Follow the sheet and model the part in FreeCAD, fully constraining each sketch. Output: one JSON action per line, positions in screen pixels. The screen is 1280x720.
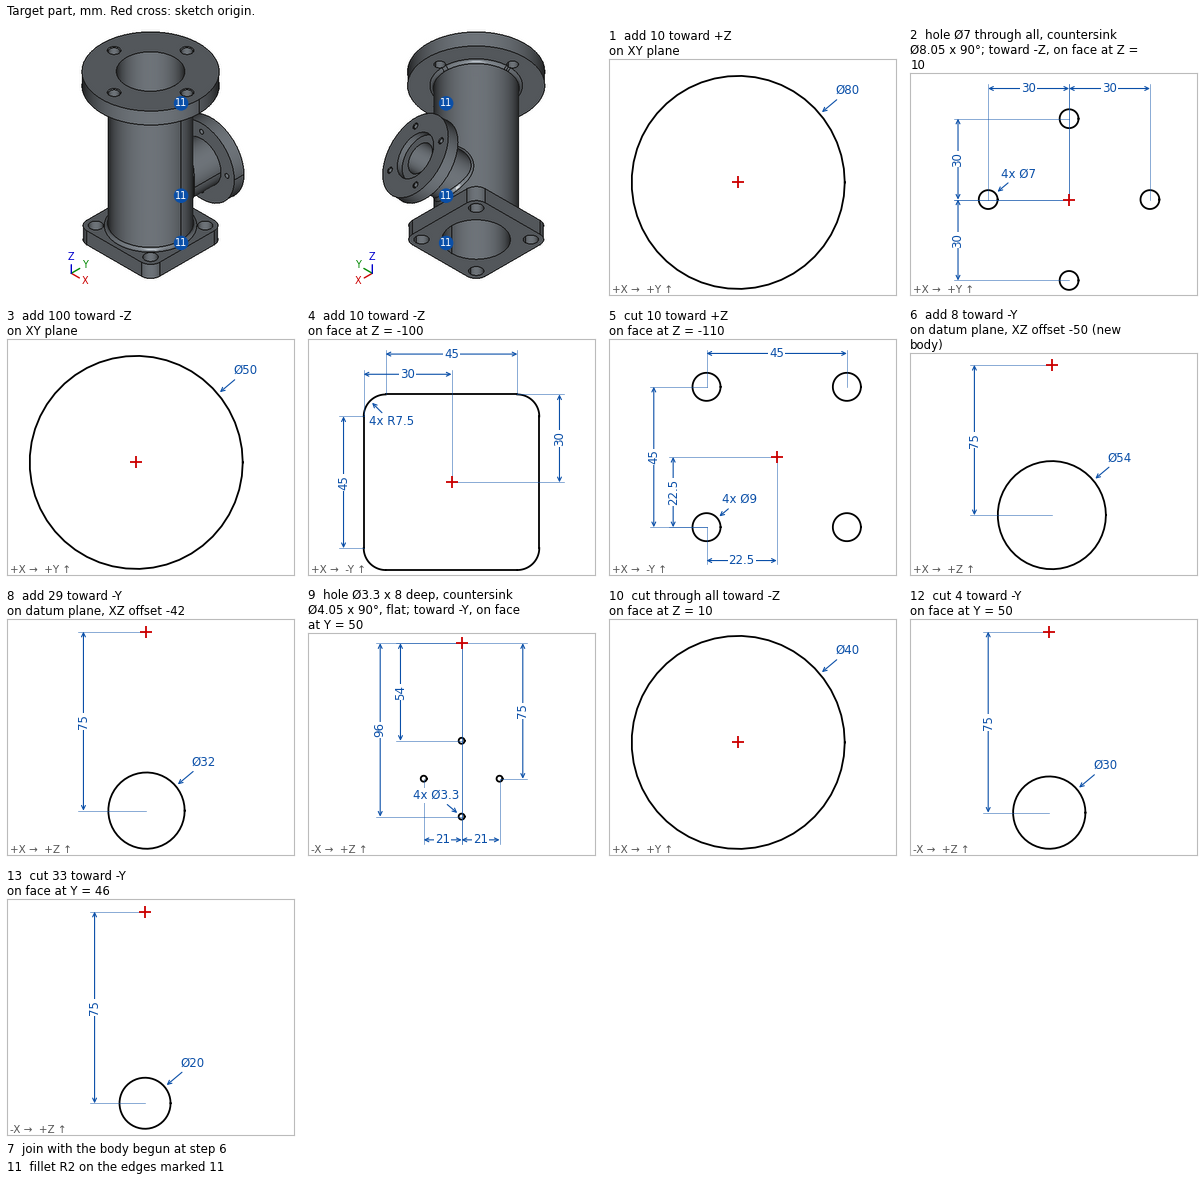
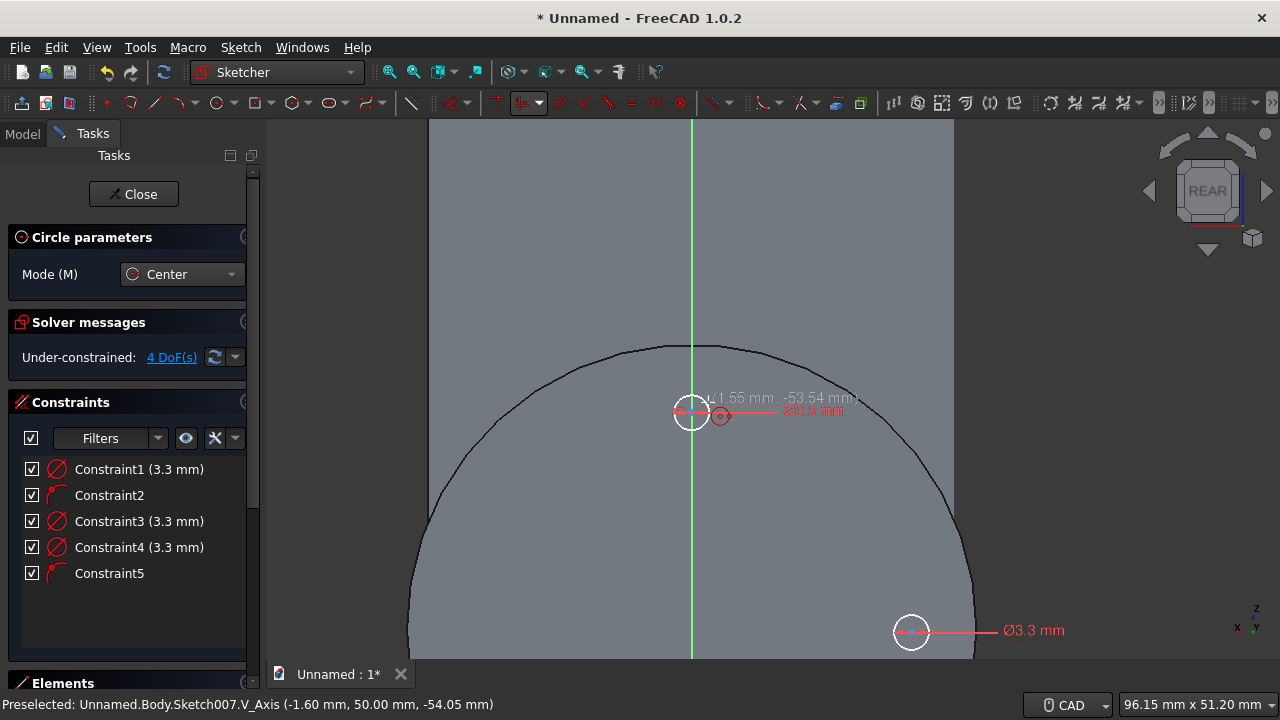
{"action": "scroll", "coordinate": [470, 629], "scroll_direction": "up", "scroll_amount": 2}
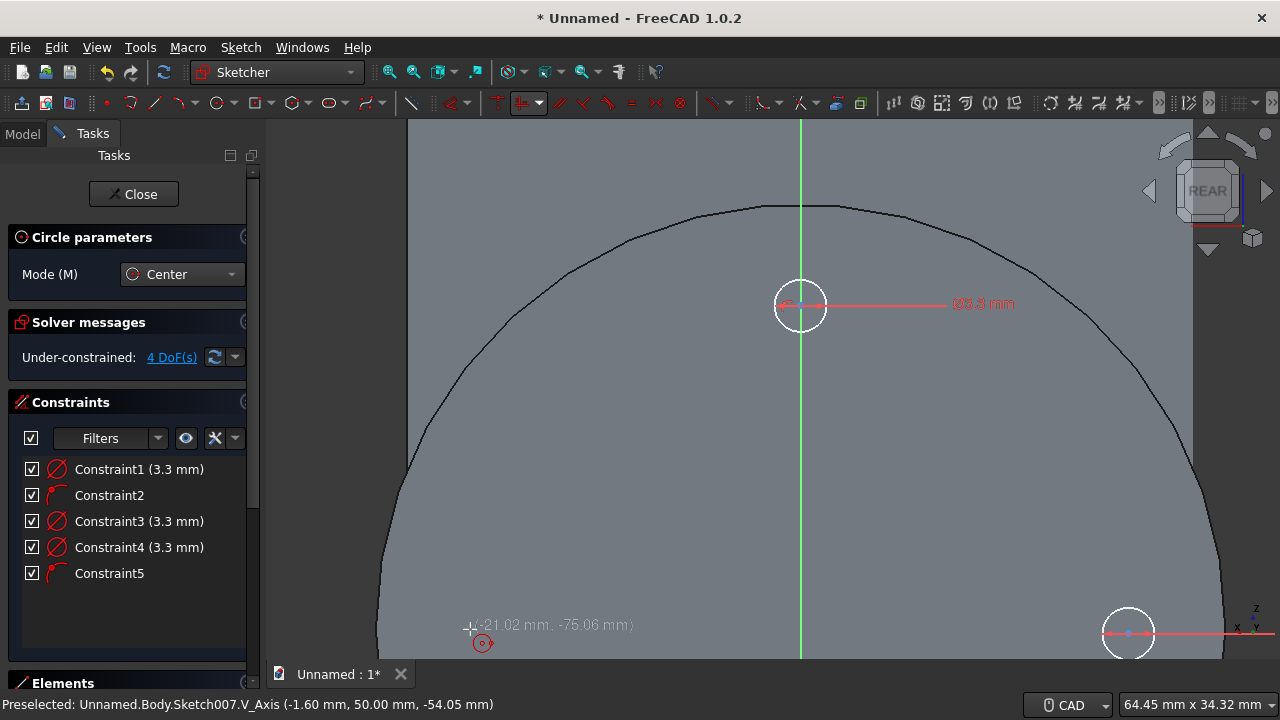
{"action": "scroll", "coordinate": [680, 432], "scroll_direction": "down", "scroll_amount": 8}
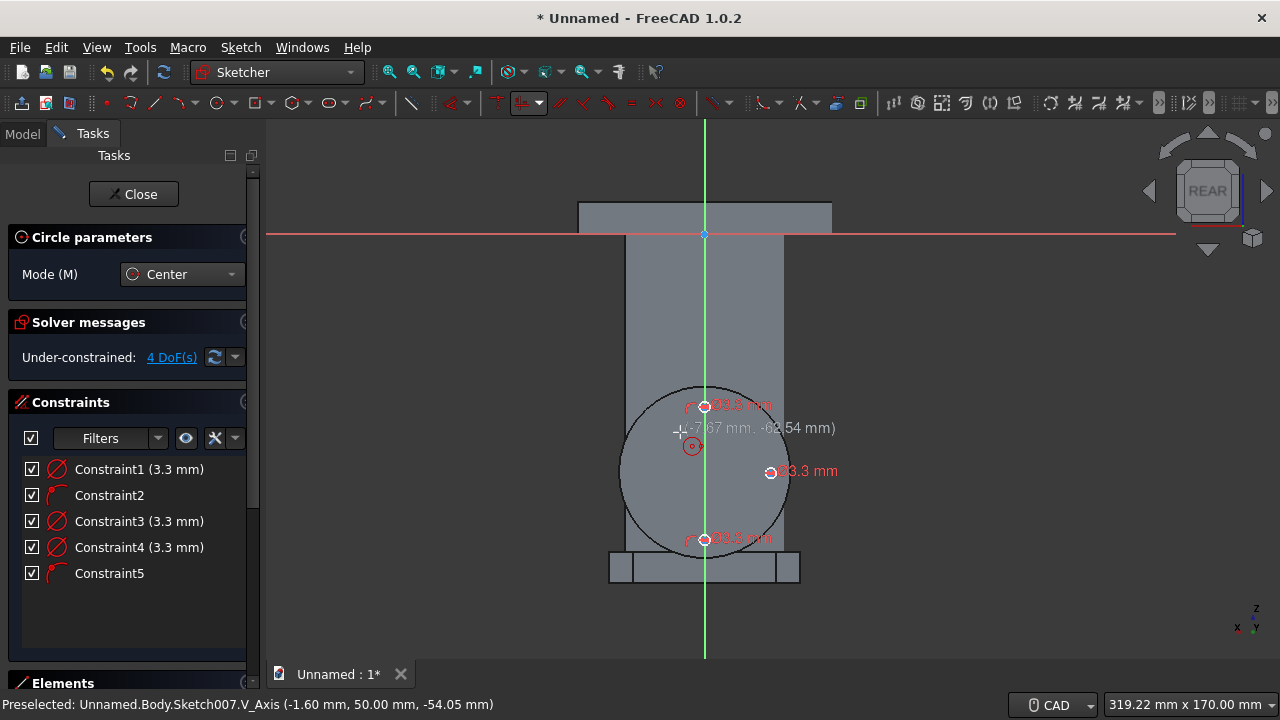
{"action": "left_click", "coordinate": [638, 472]}
{"action": "mouse_move", "coordinate": [642, 469]}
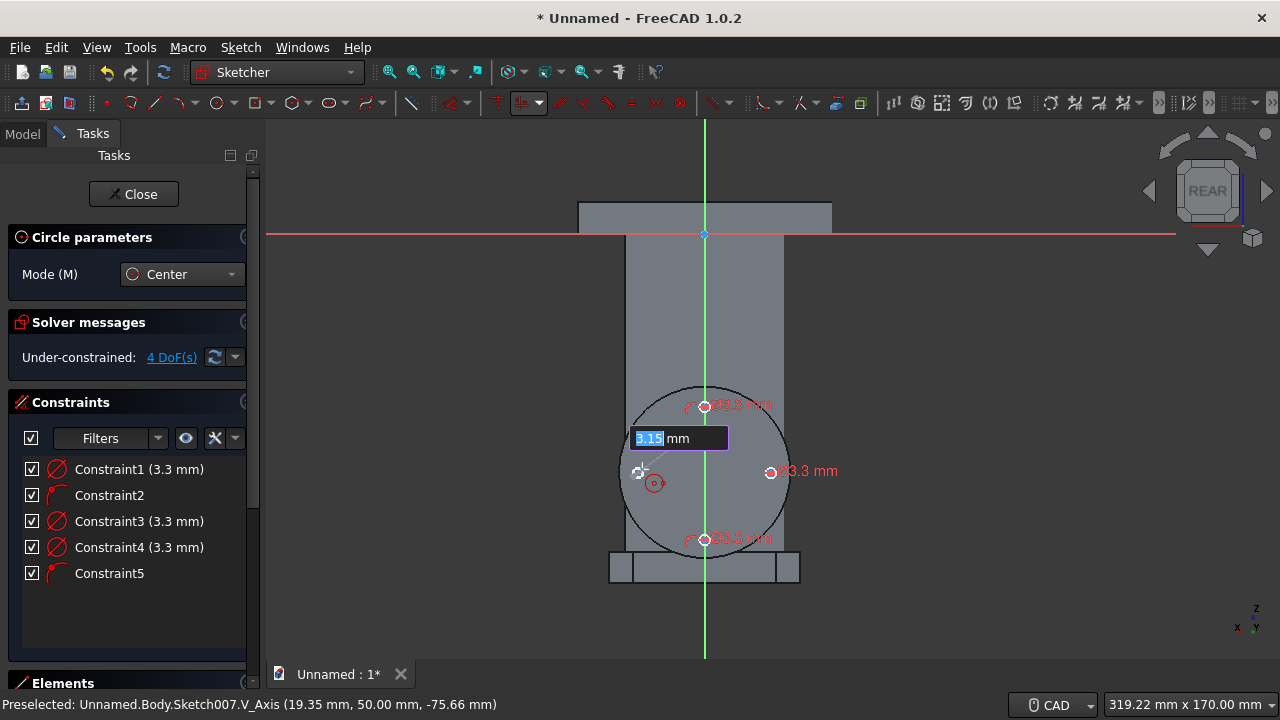
{"action": "type", "text": "3.3"}
{"action": "key", "text": "Return"}
{"action": "key", "text": "Escape"}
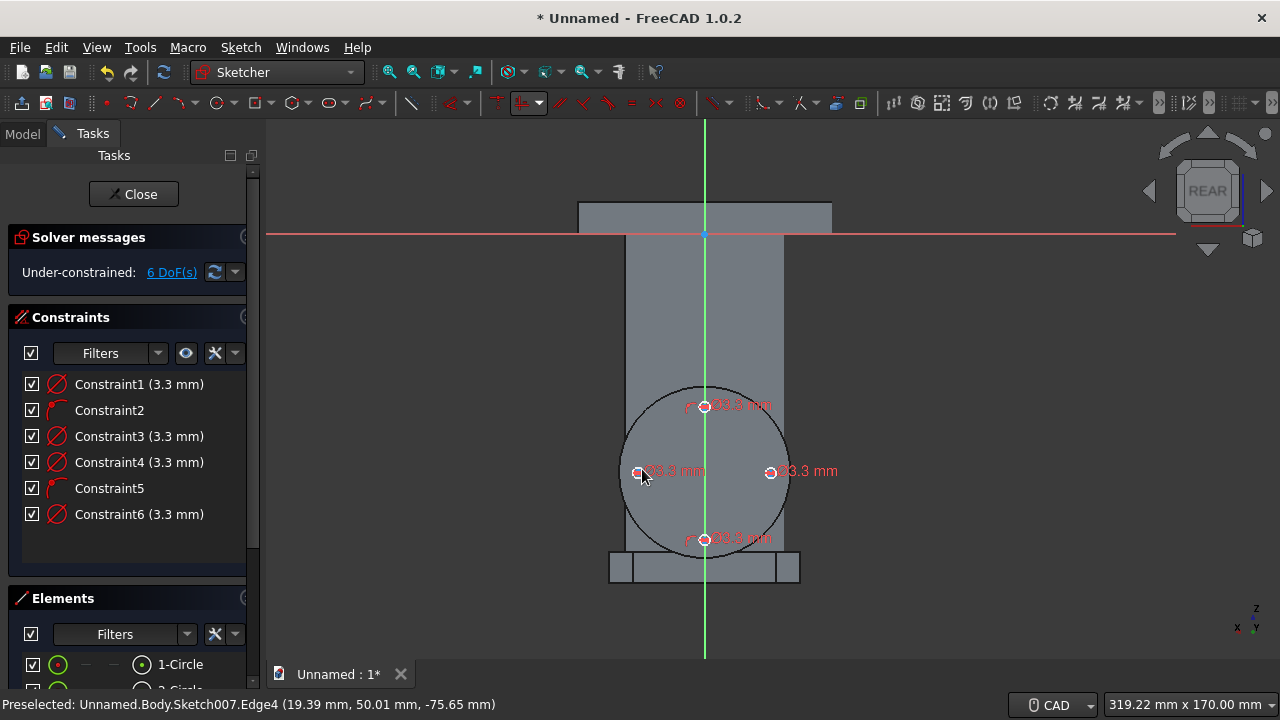
{"action": "left_click", "coordinate": [771, 473]}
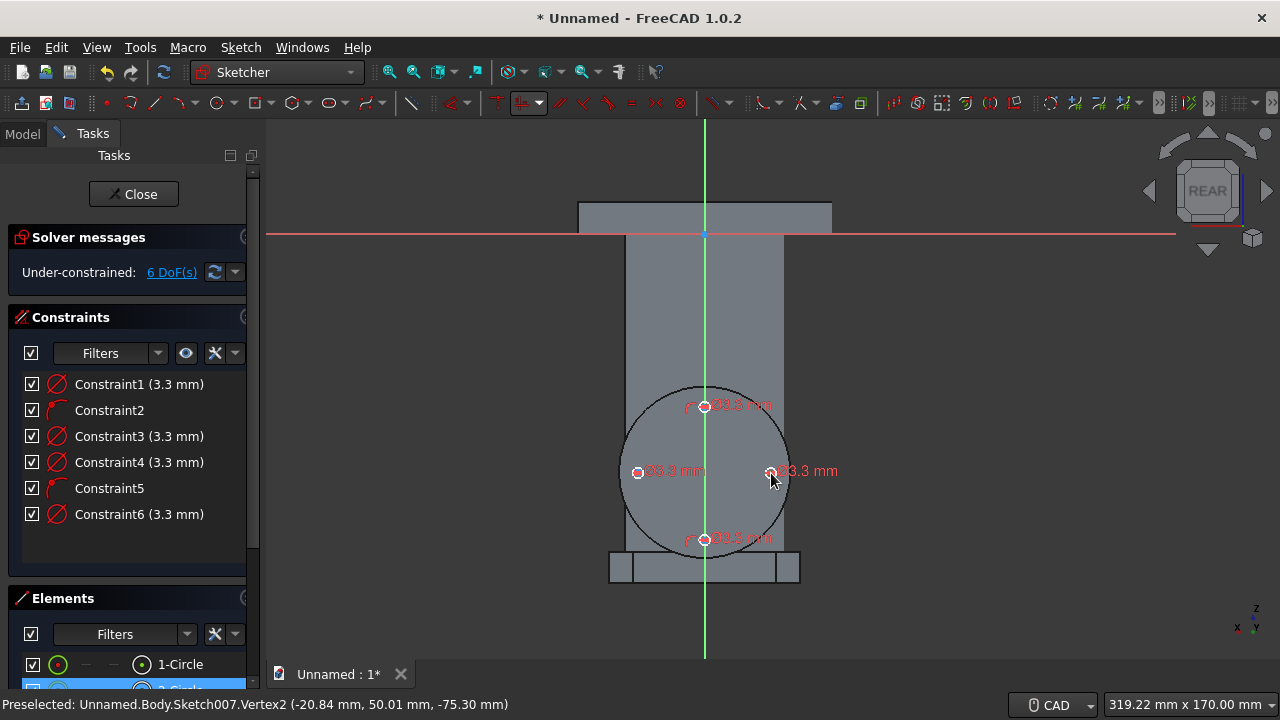
{"action": "left_click", "coordinate": [638, 473]}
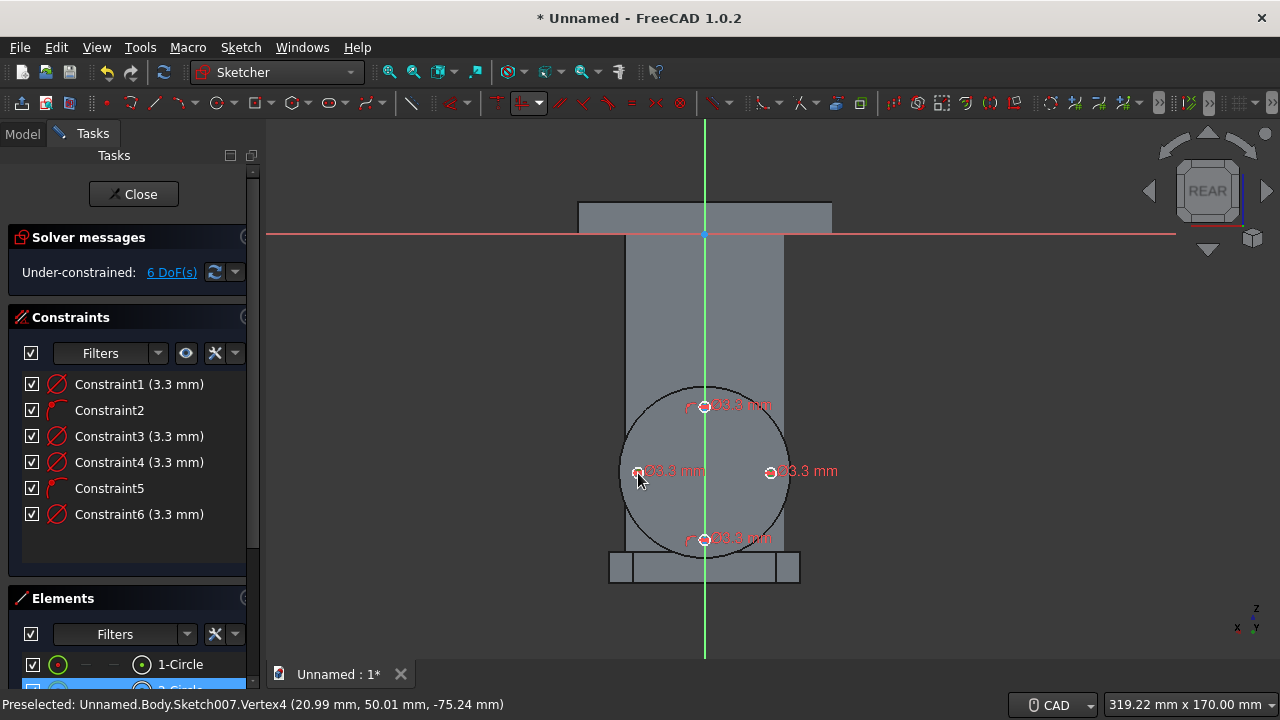
{"action": "key", "text": "h"}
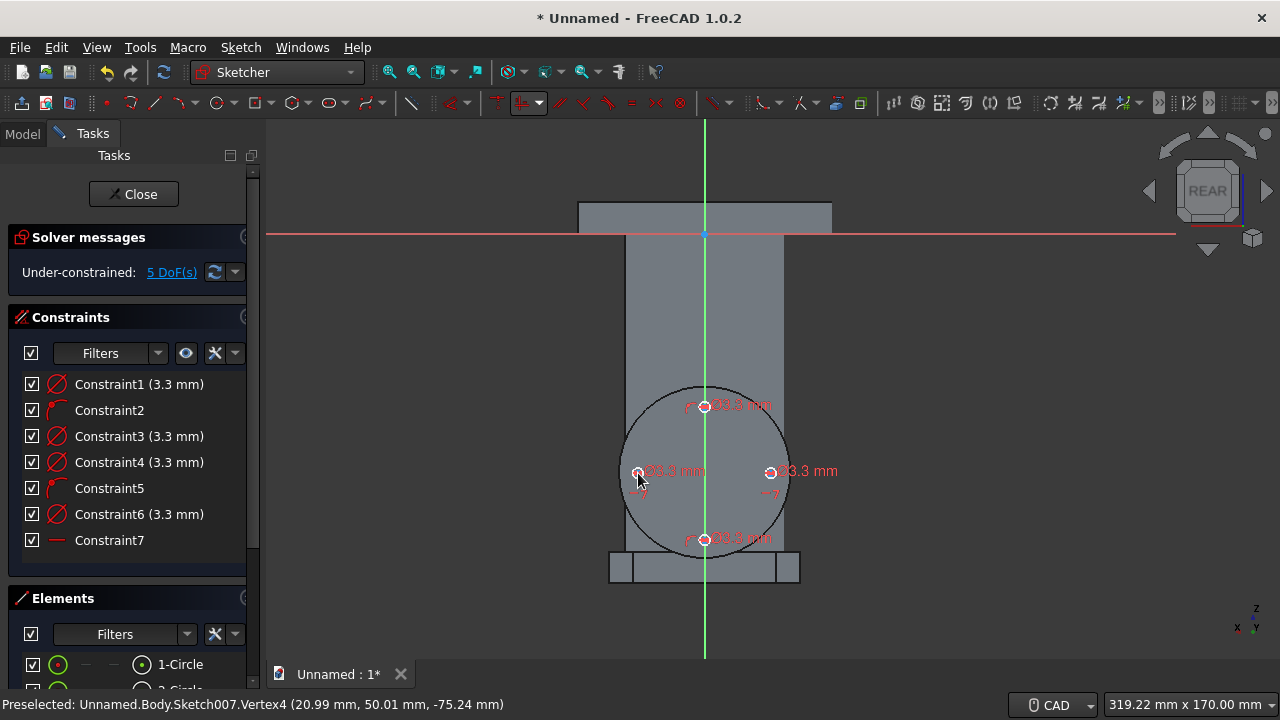
{"action": "left_click", "coordinate": [450, 104]}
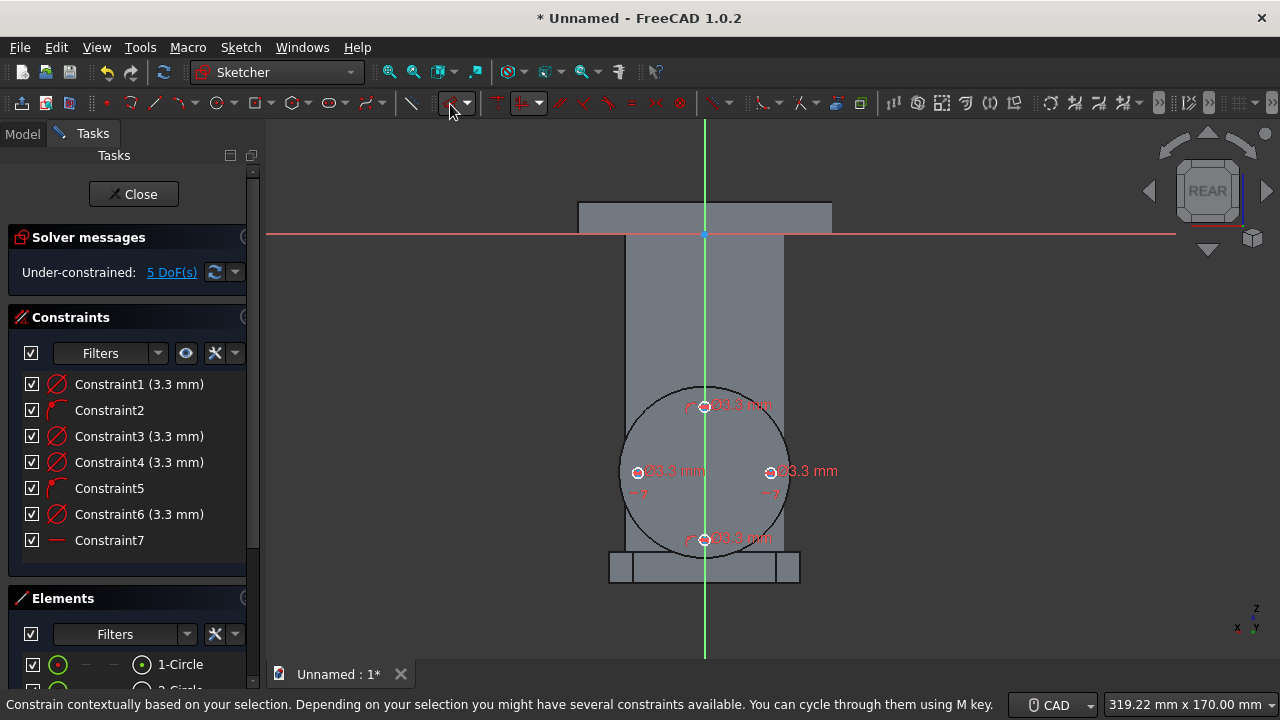
{"action": "left_click", "coordinate": [705, 540]}
{"action": "left_click", "coordinate": [739, 387]}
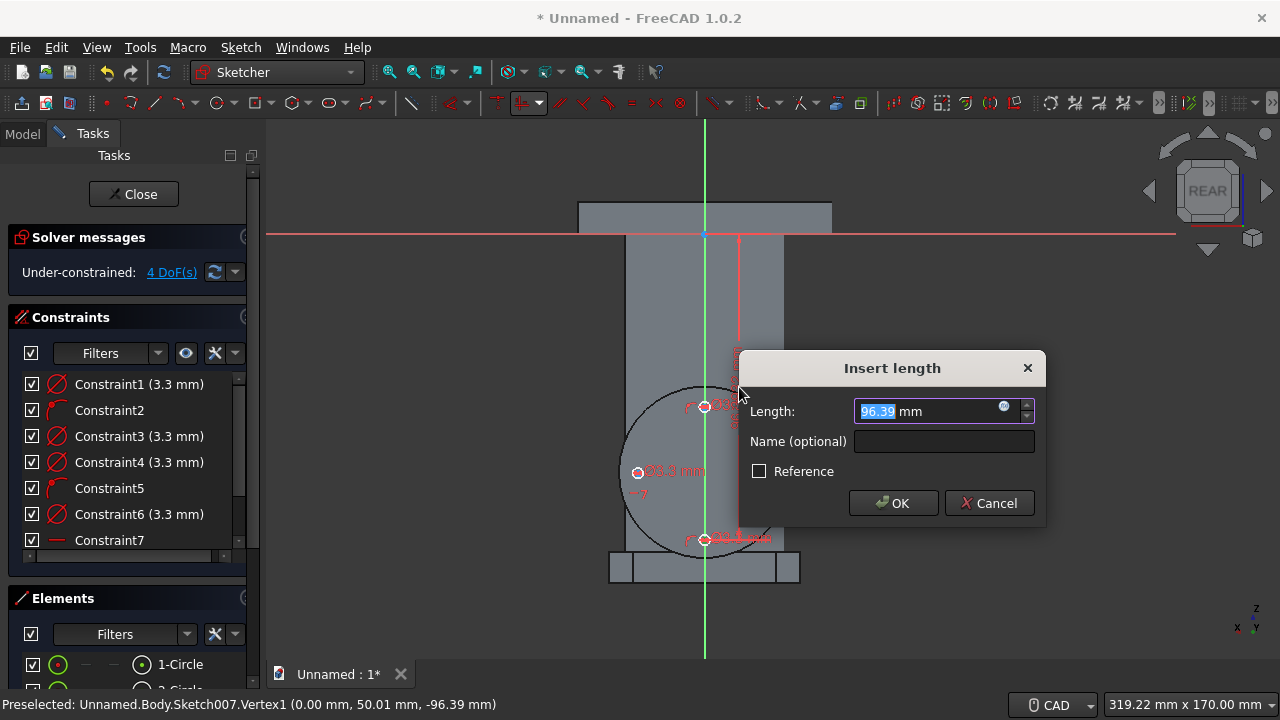
{"action": "type", "text": "96"}
{"action": "key", "text": "Return"}